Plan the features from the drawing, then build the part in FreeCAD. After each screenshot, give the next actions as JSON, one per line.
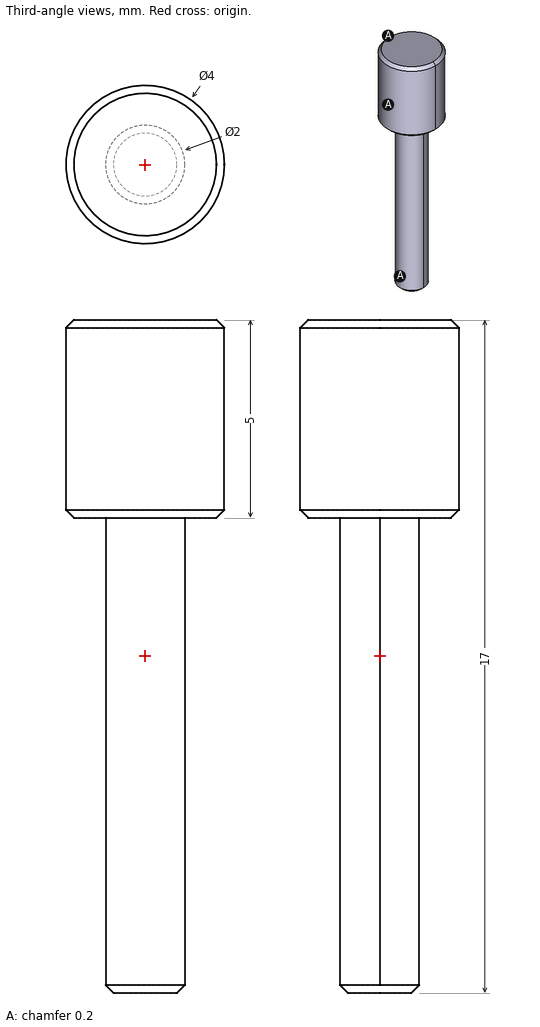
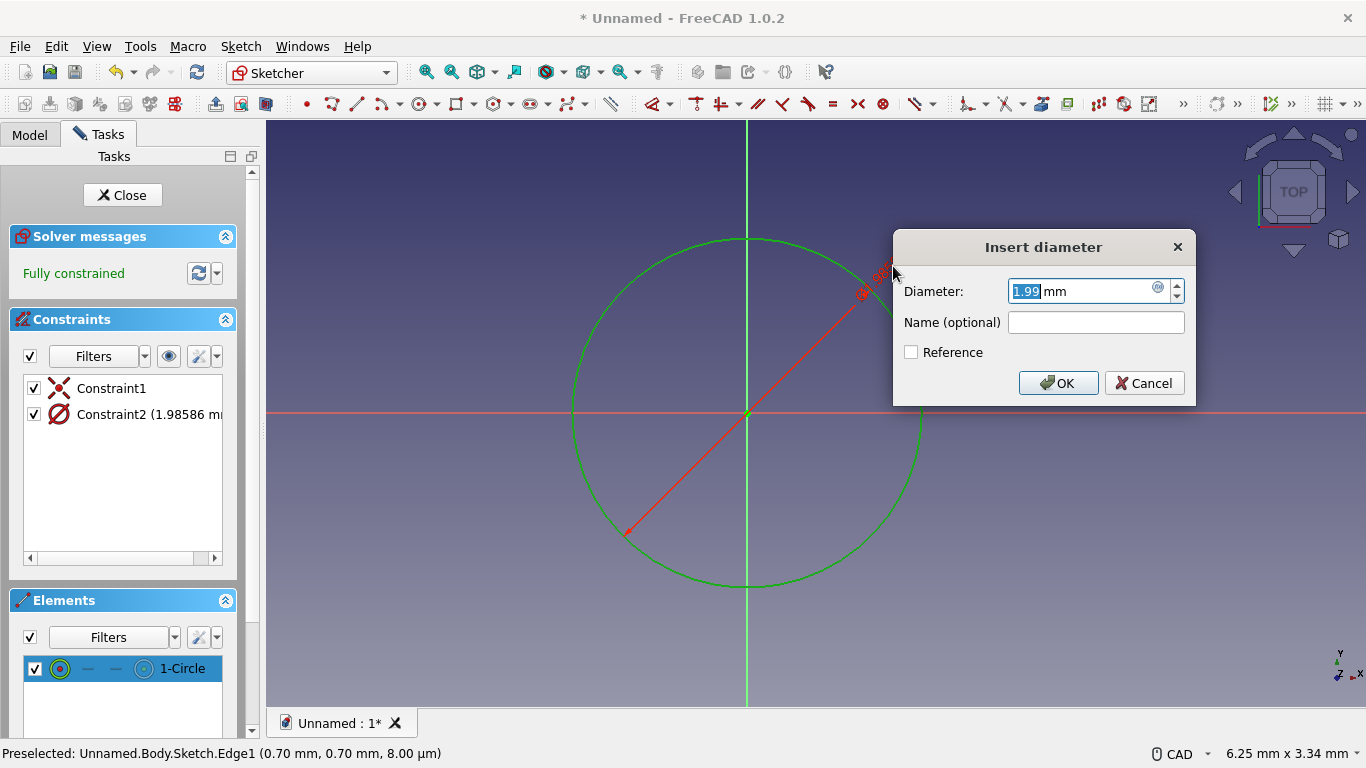
{"action": "type", "text": "2"}
{"action": "key", "text": "Return"}
{"action": "key", "text": "Escape"}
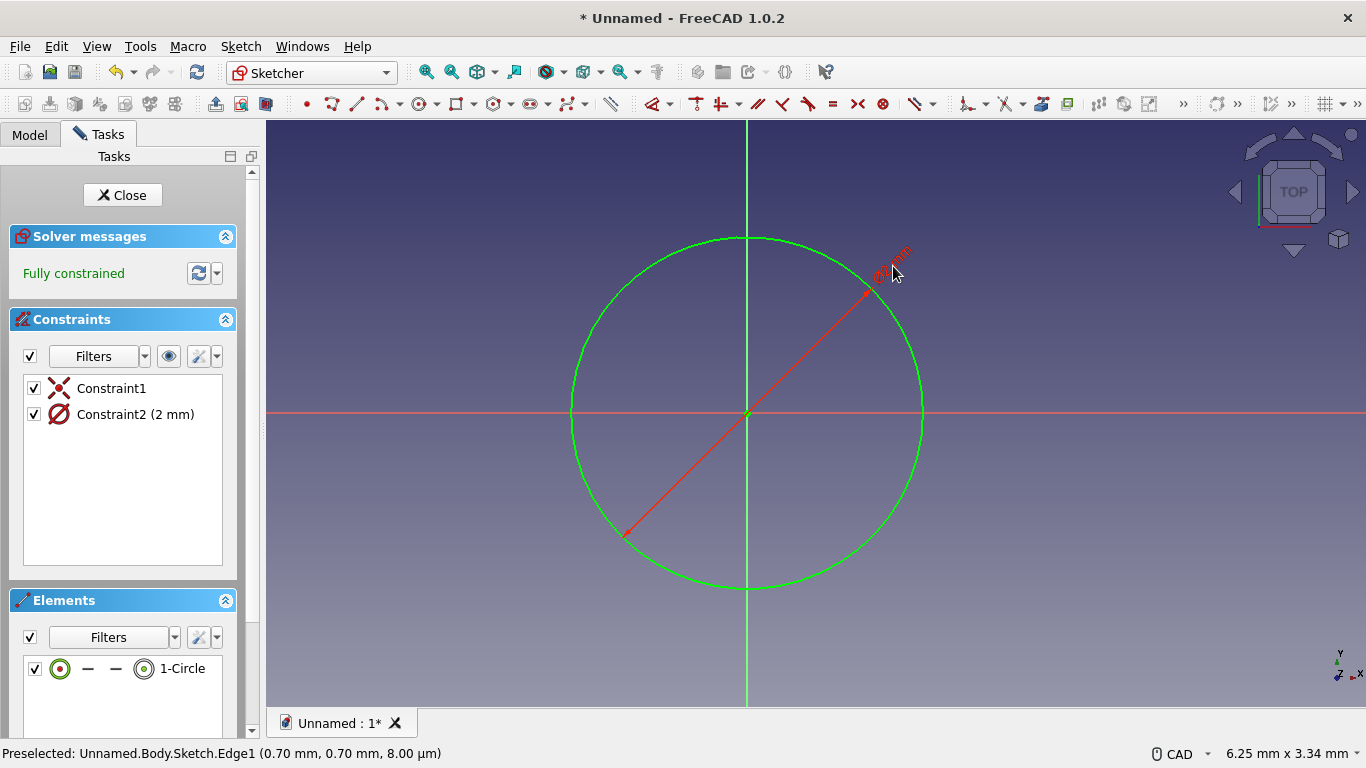
{"action": "left_click", "coordinate": [123, 195]}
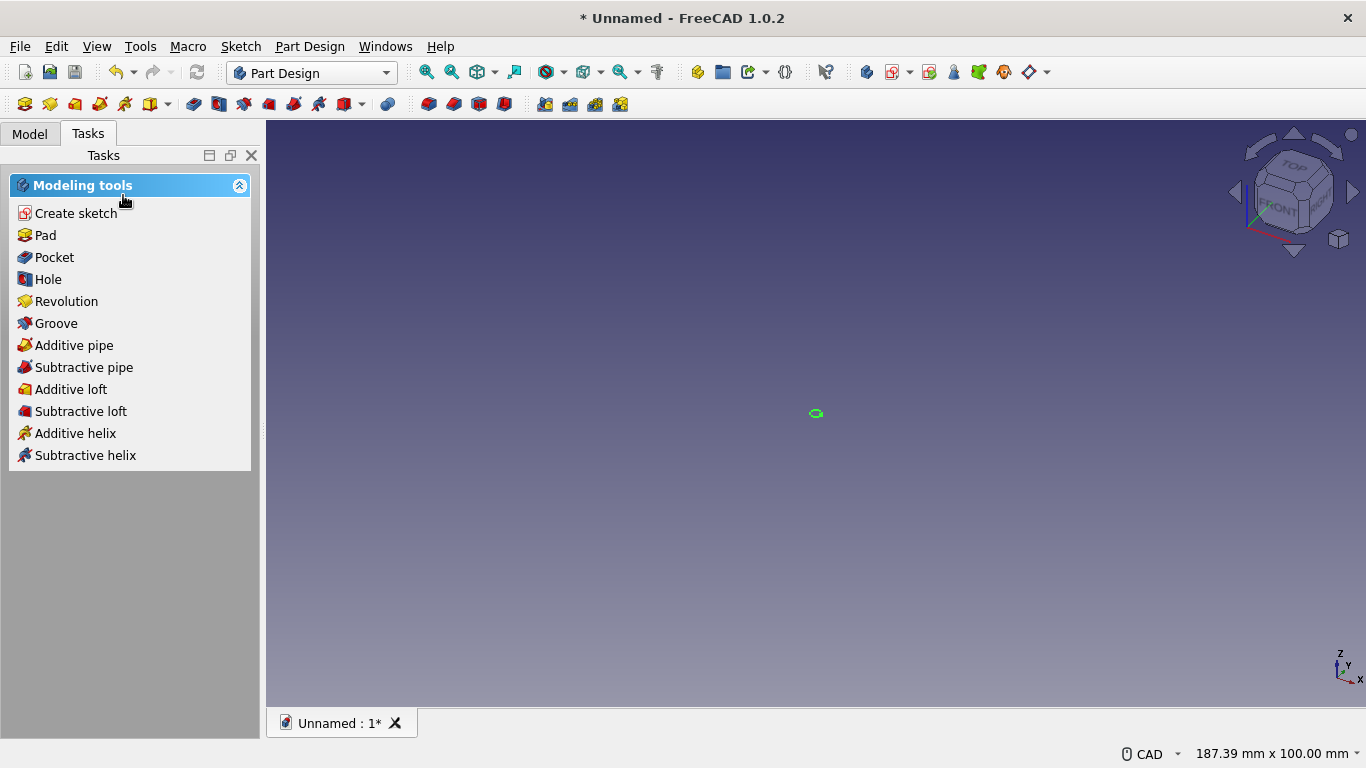
{"action": "left_click", "coordinate": [25, 104]}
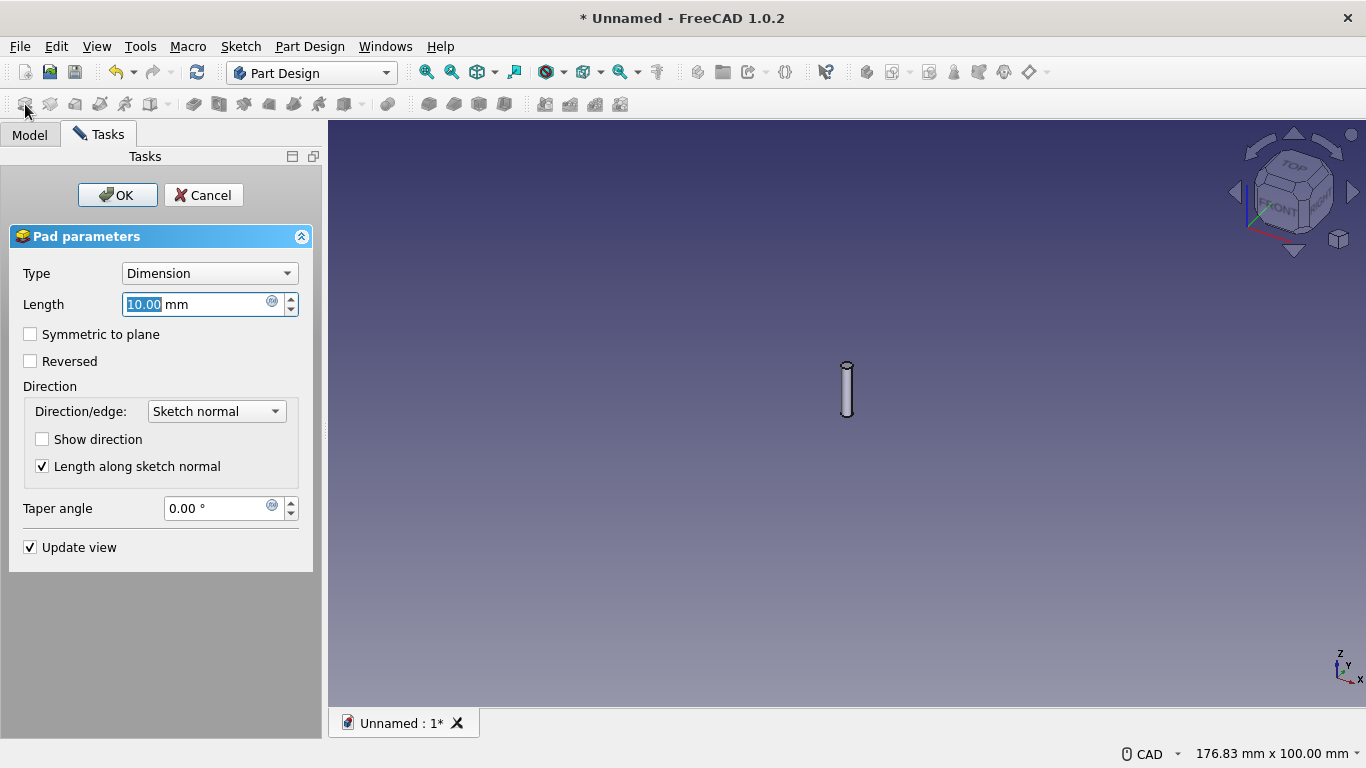
{"action": "type", "text": "17"}
{"action": "key", "text": "Tab"}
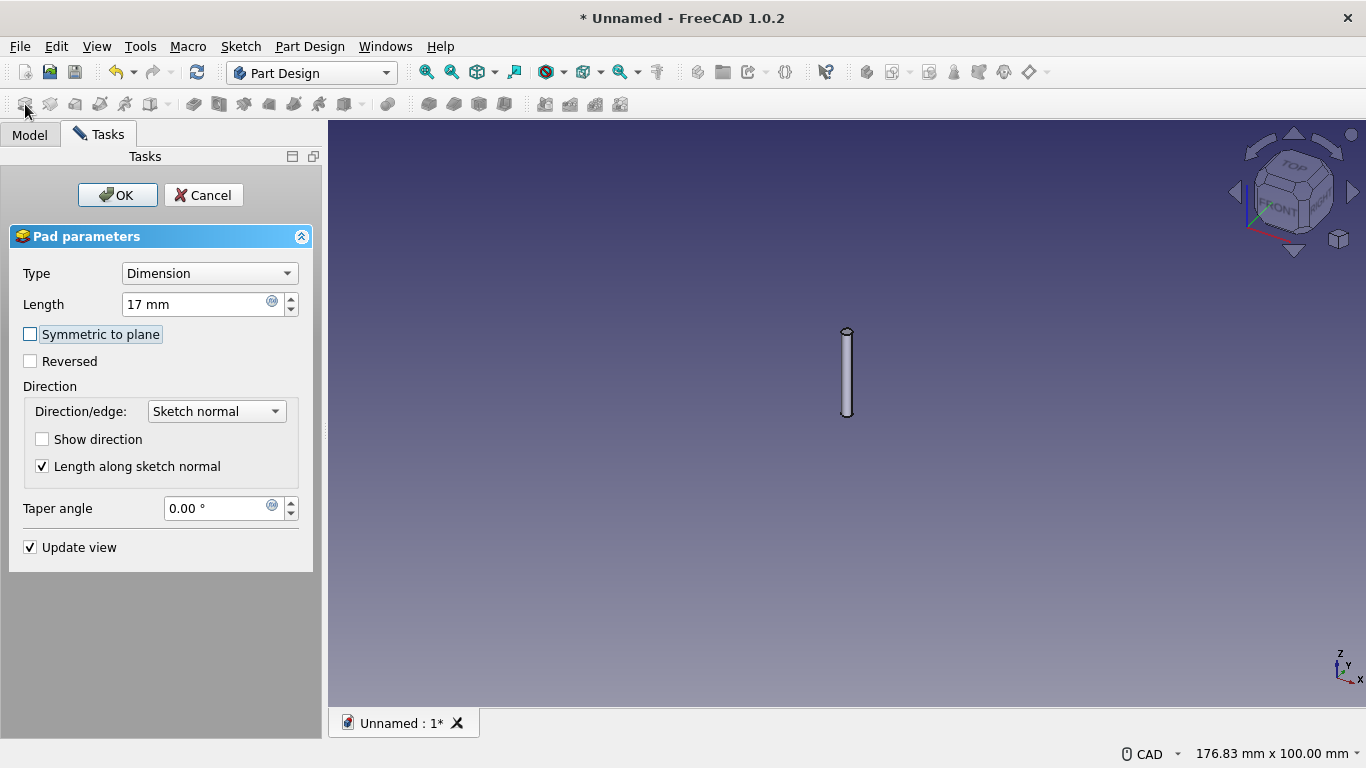
{"action": "left_click", "coordinate": [31, 334]}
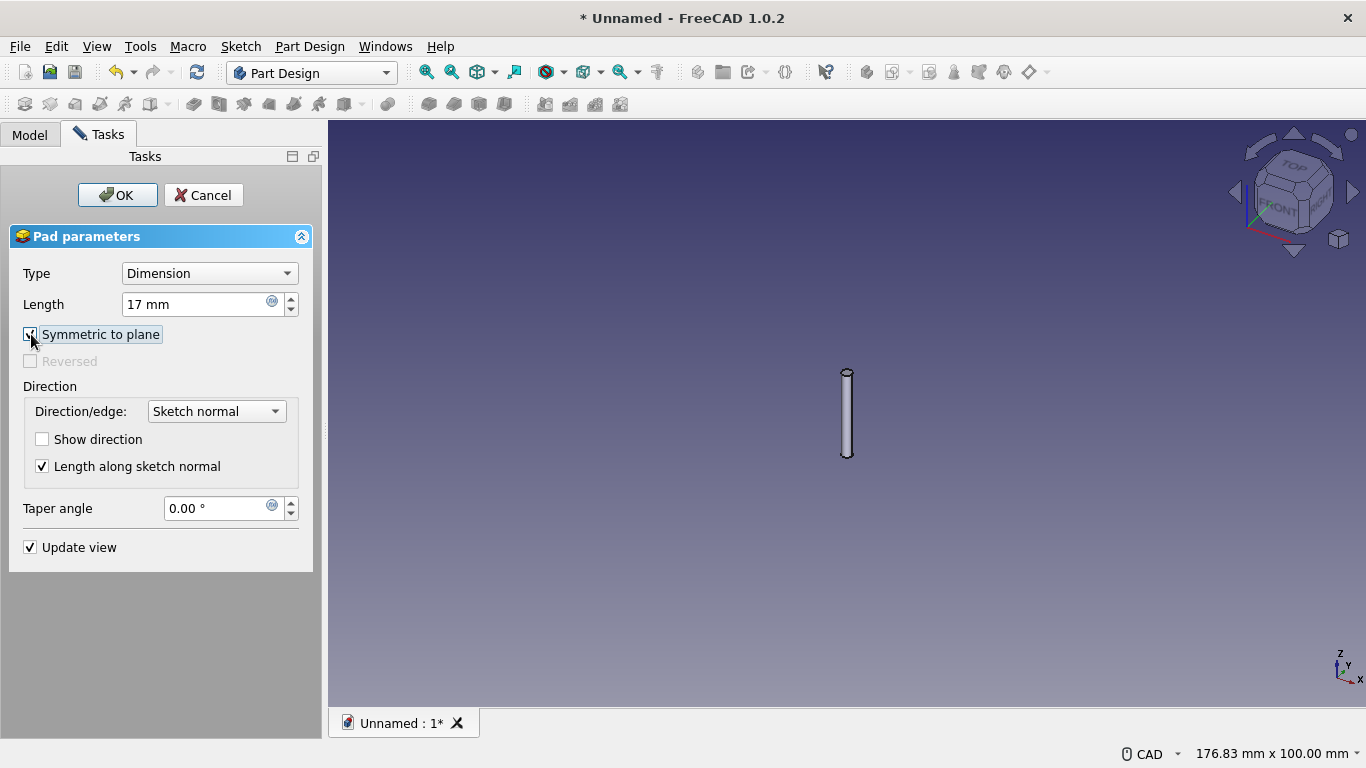
{"action": "left_click", "coordinate": [118, 195]}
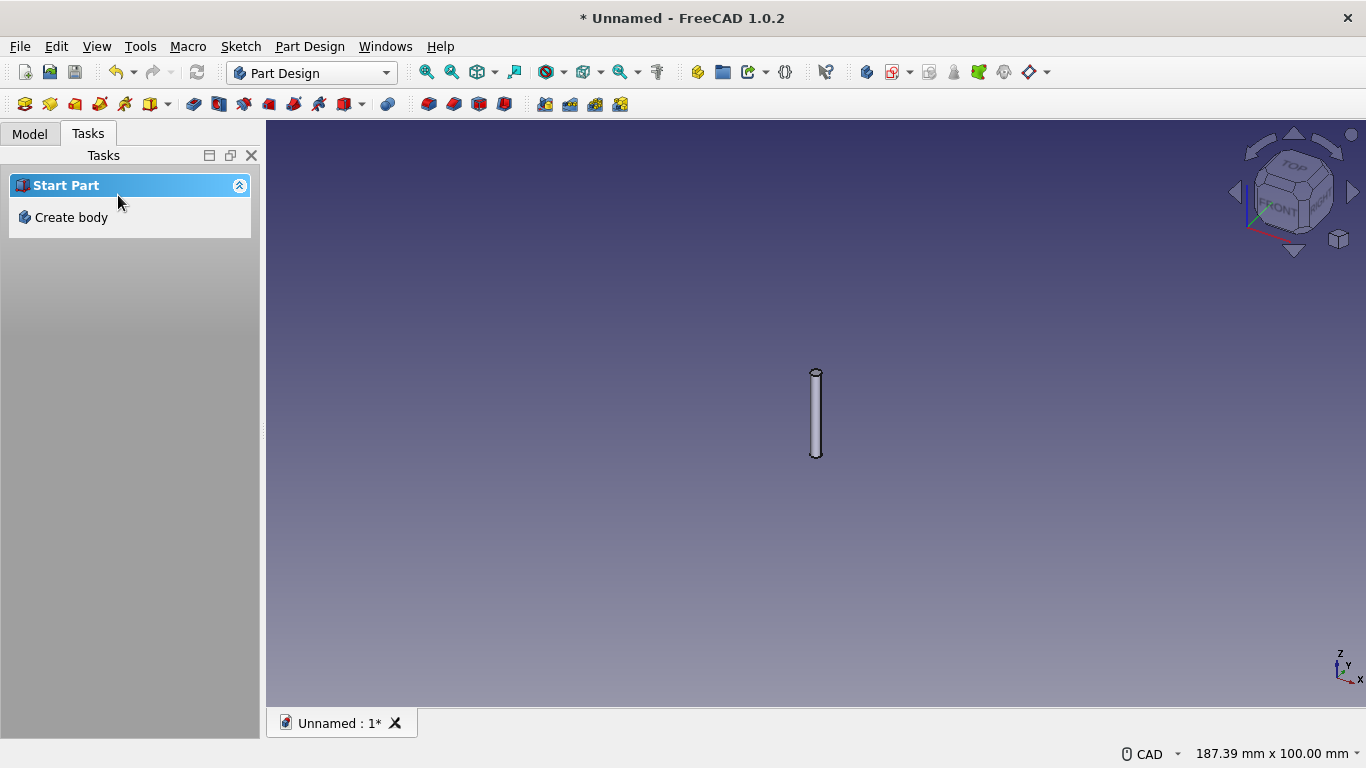
{"action": "left_click", "coordinate": [427, 72]}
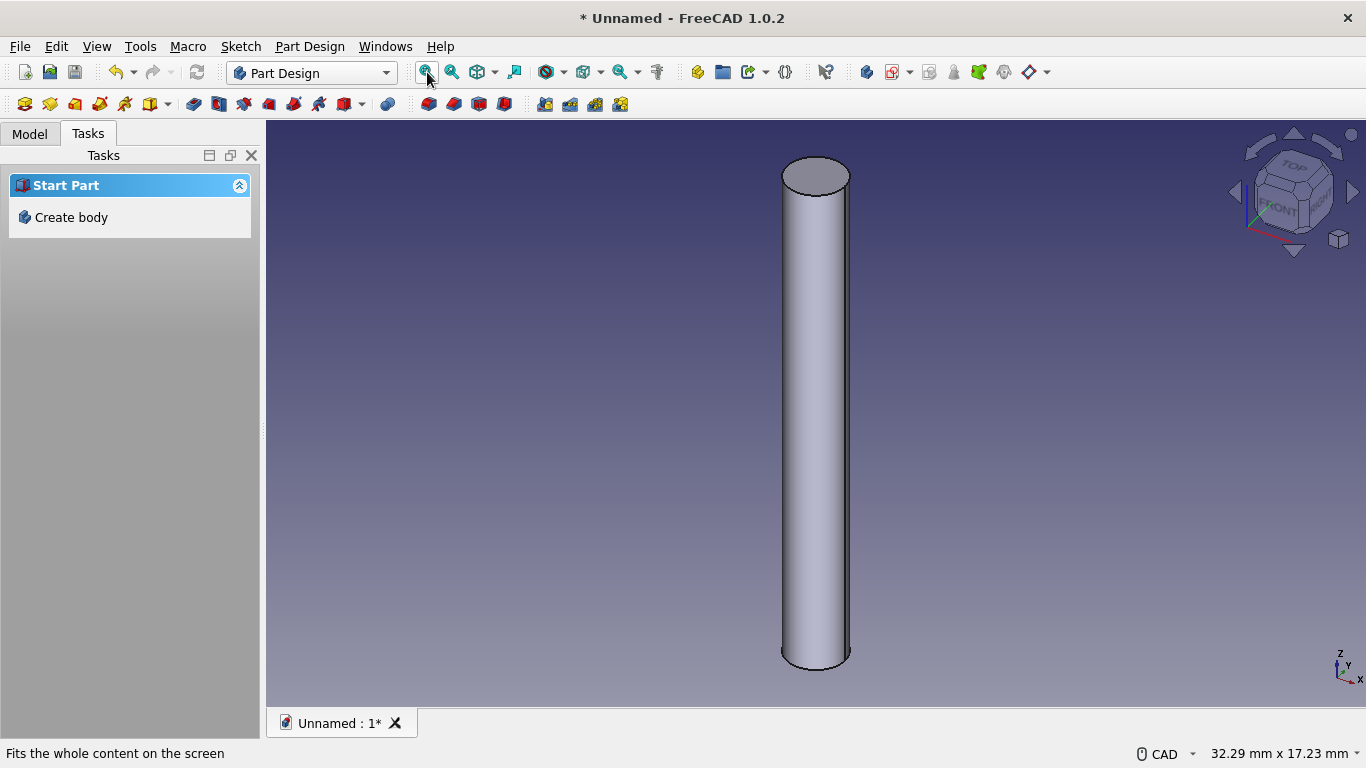
{"action": "left_click", "coordinate": [816, 175]}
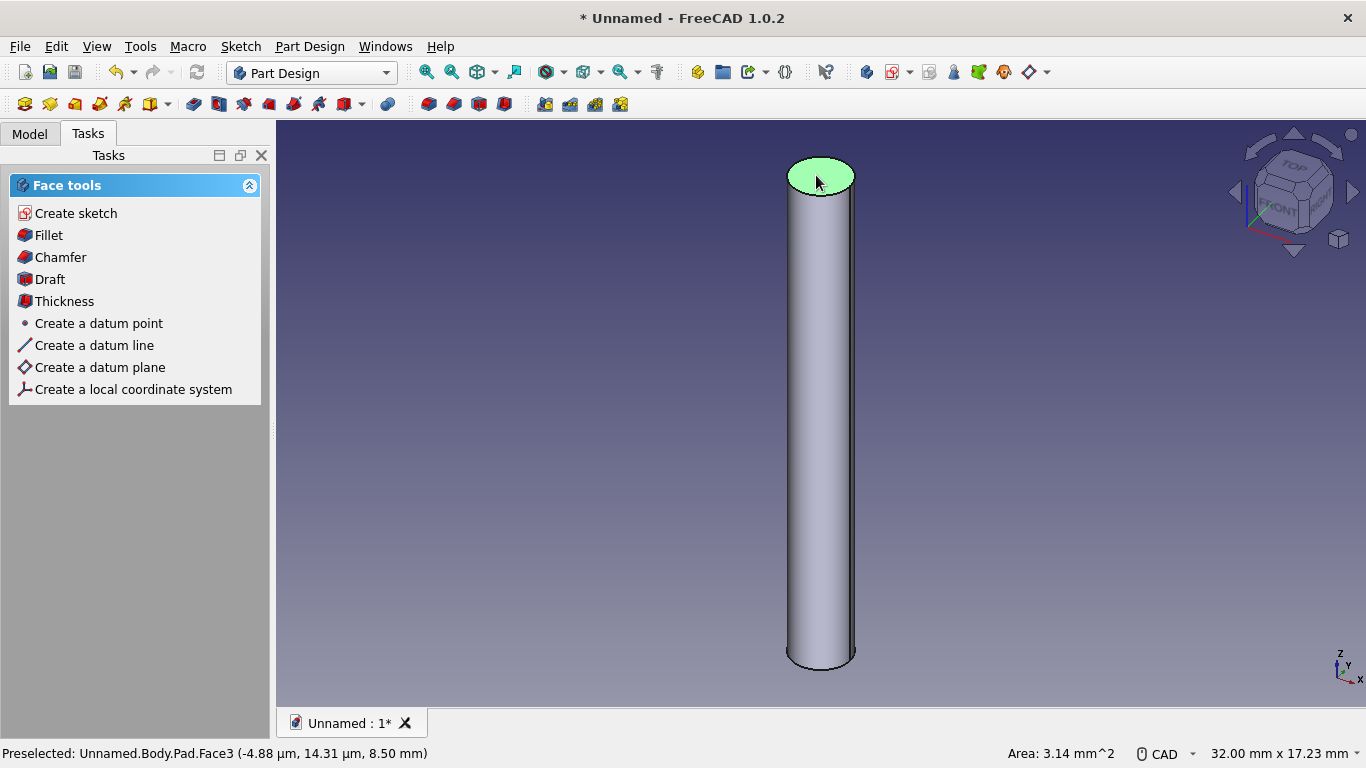
{"action": "left_click", "coordinate": [892, 72]}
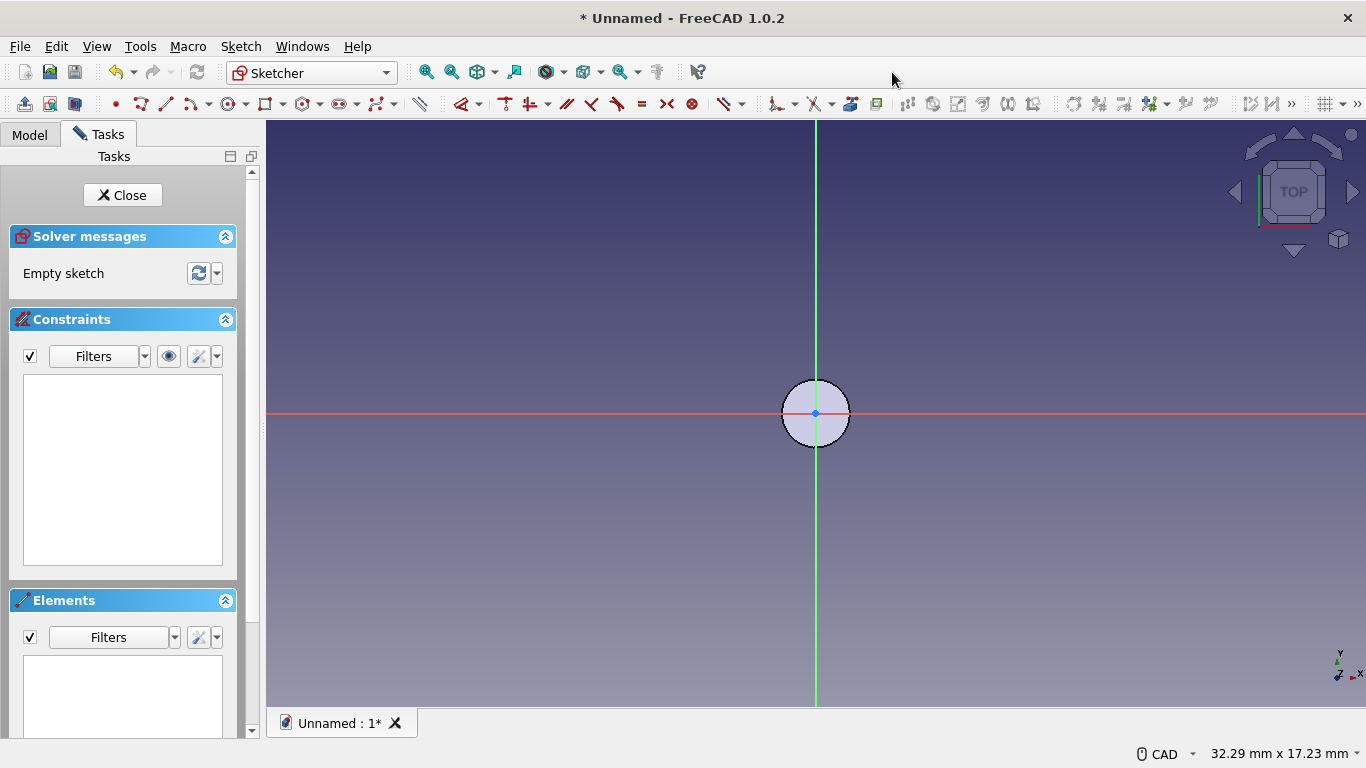
{"action": "scroll", "coordinate": [856, 414], "scroll_direction": "up", "scroll_amount": 5}